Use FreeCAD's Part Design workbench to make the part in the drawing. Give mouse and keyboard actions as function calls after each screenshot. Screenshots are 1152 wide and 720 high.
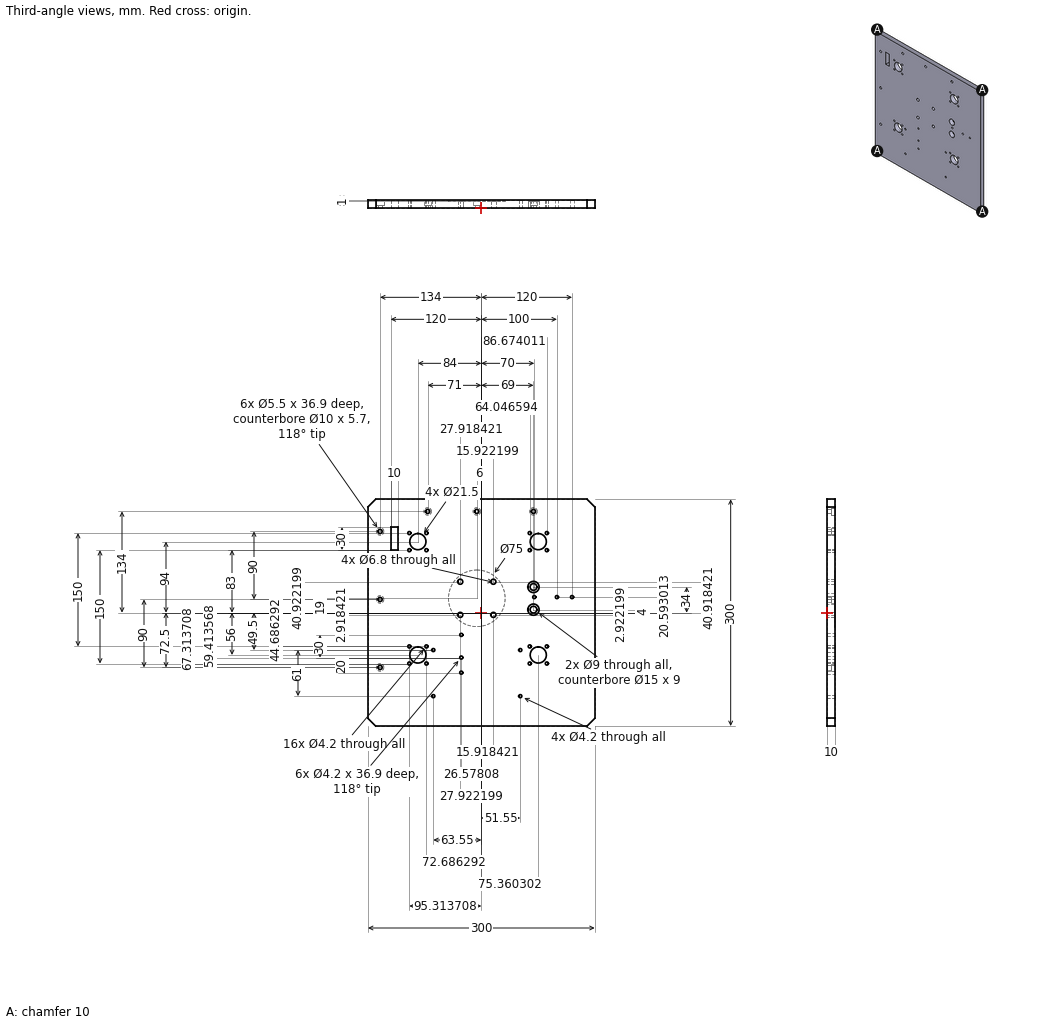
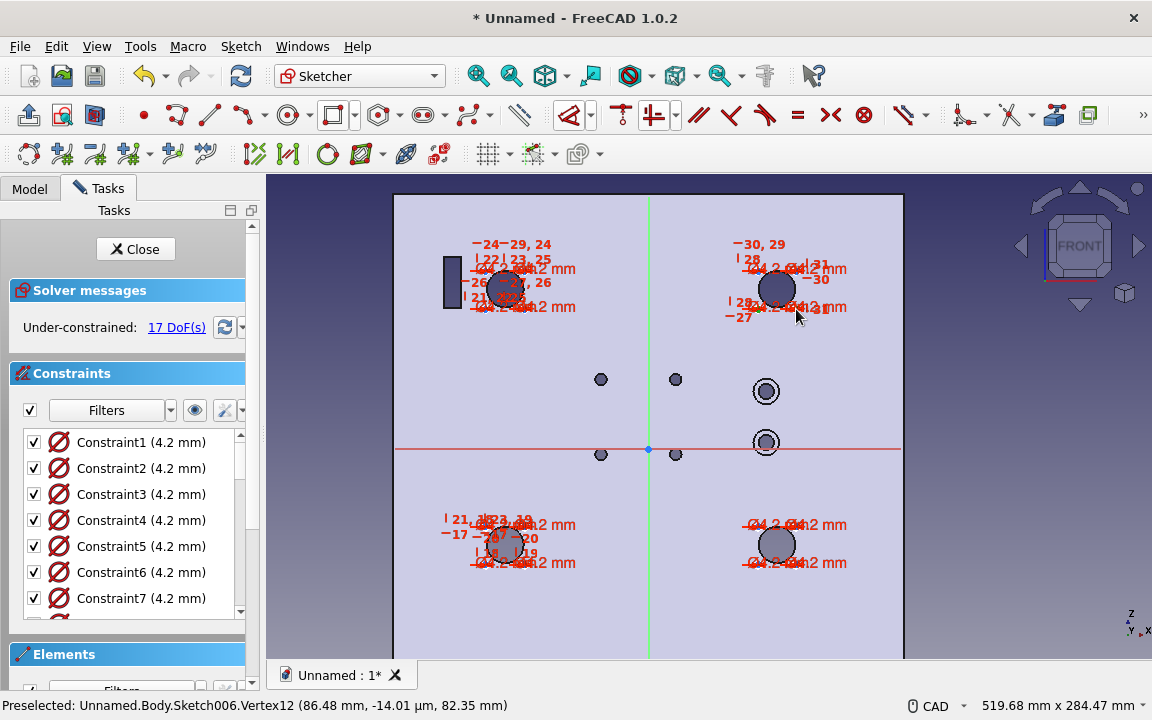
key(h)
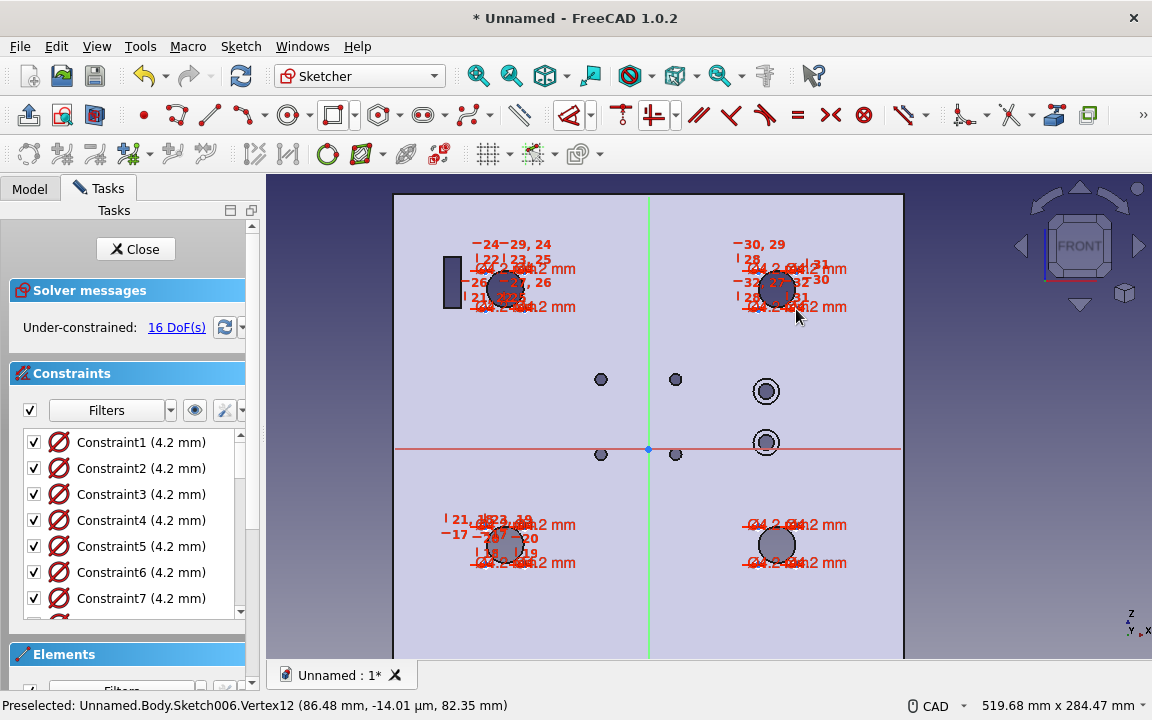
click(758, 309)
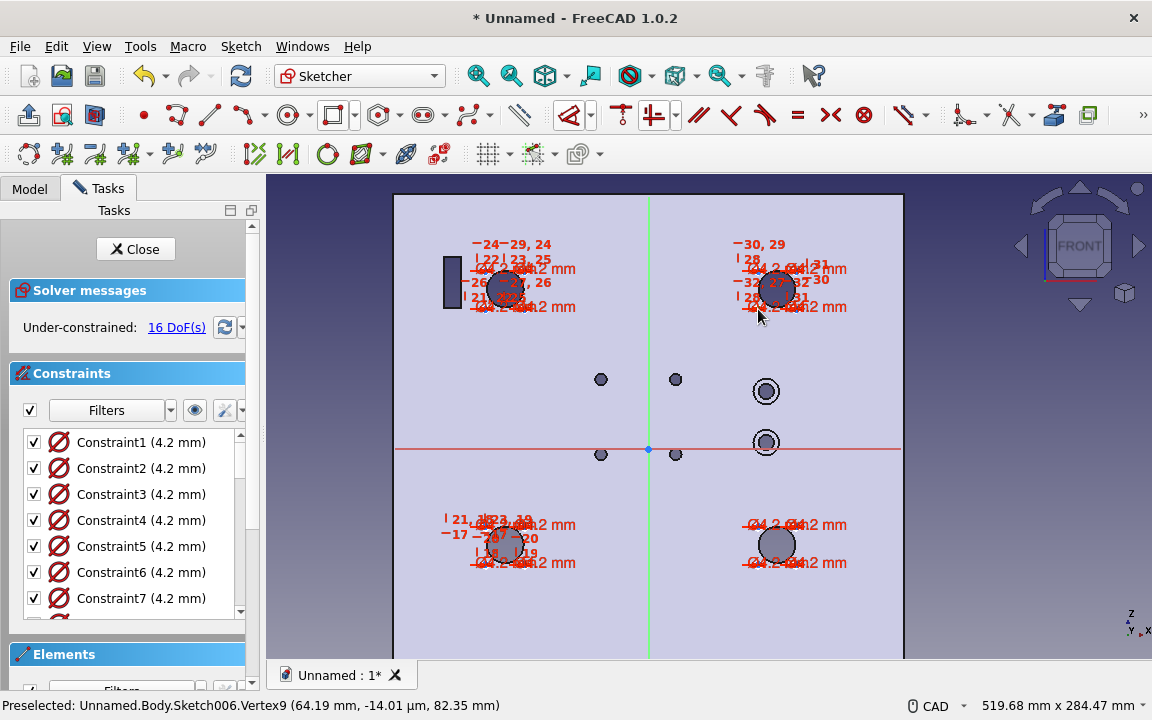
click(758, 565)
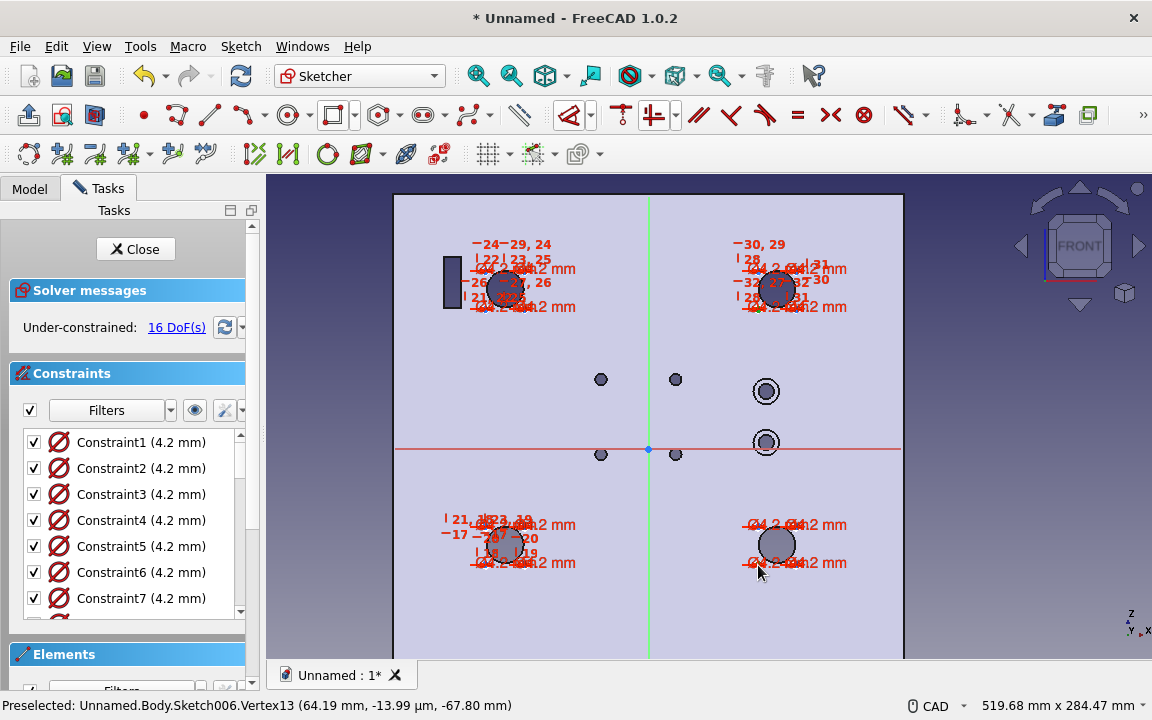
key(v)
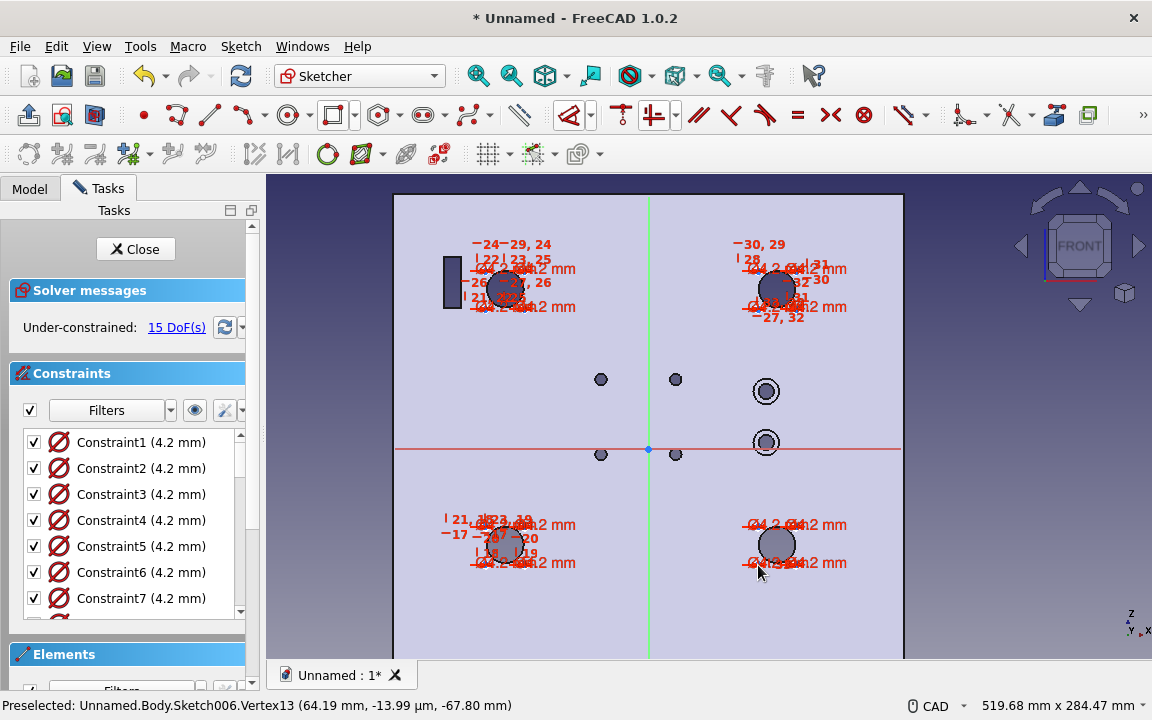
click(525, 565)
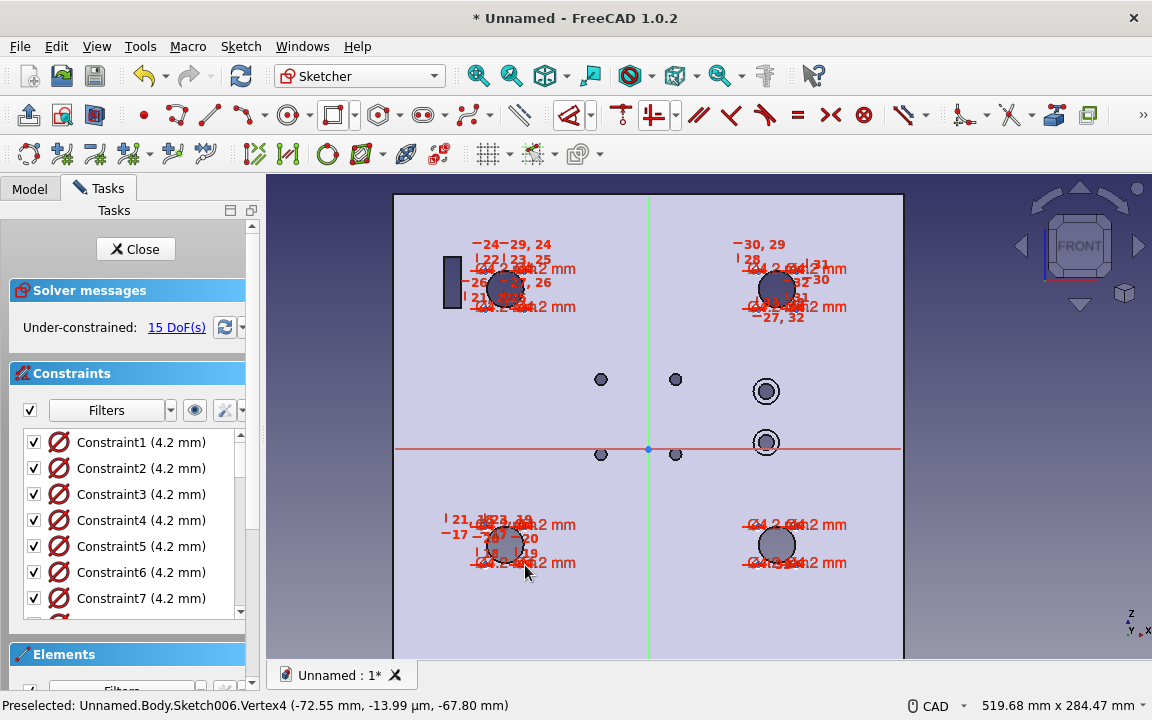
click(758, 565)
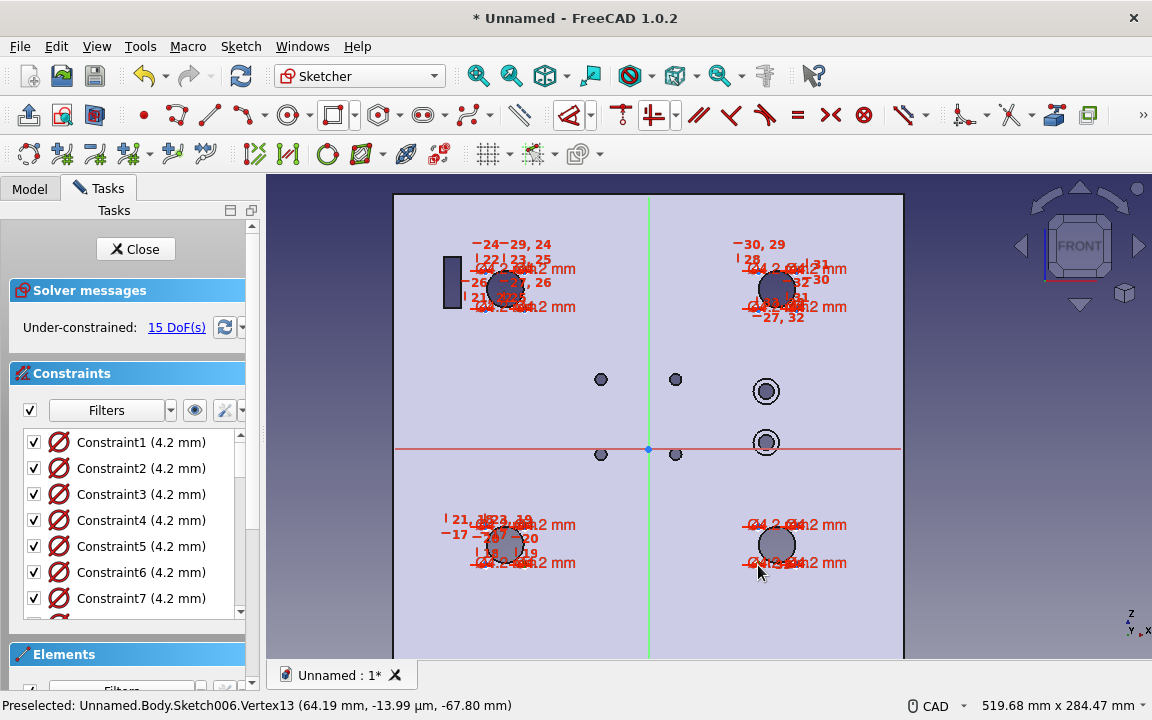
key(h)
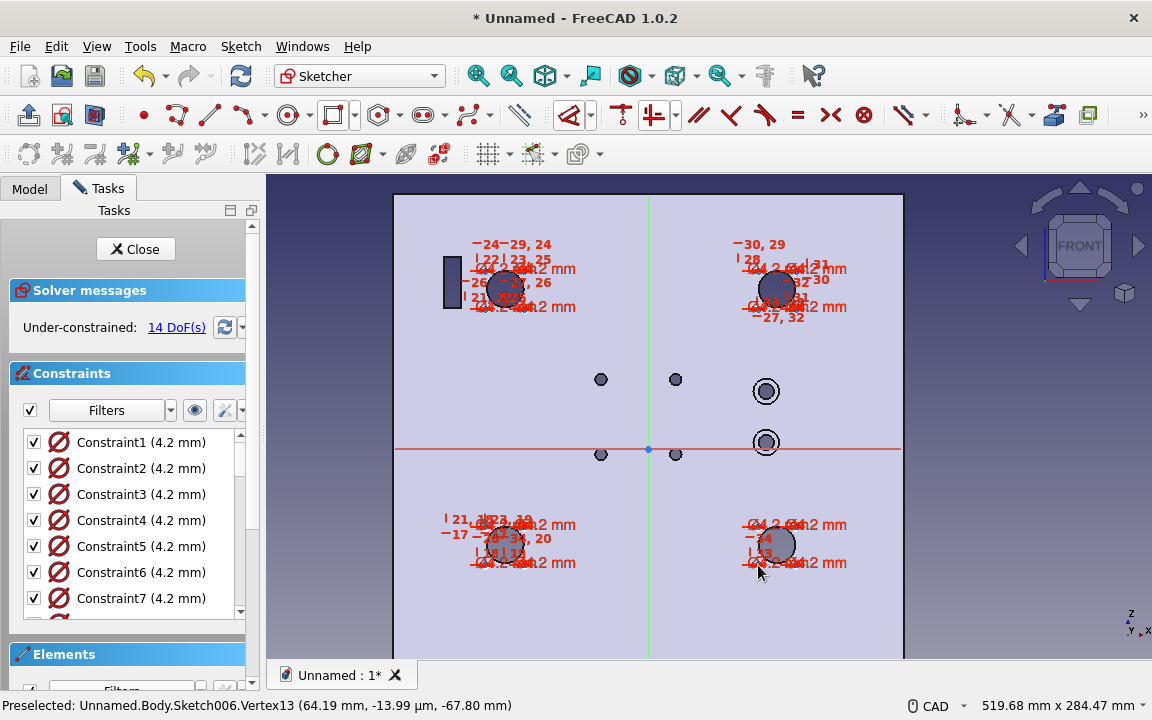
click(758, 565)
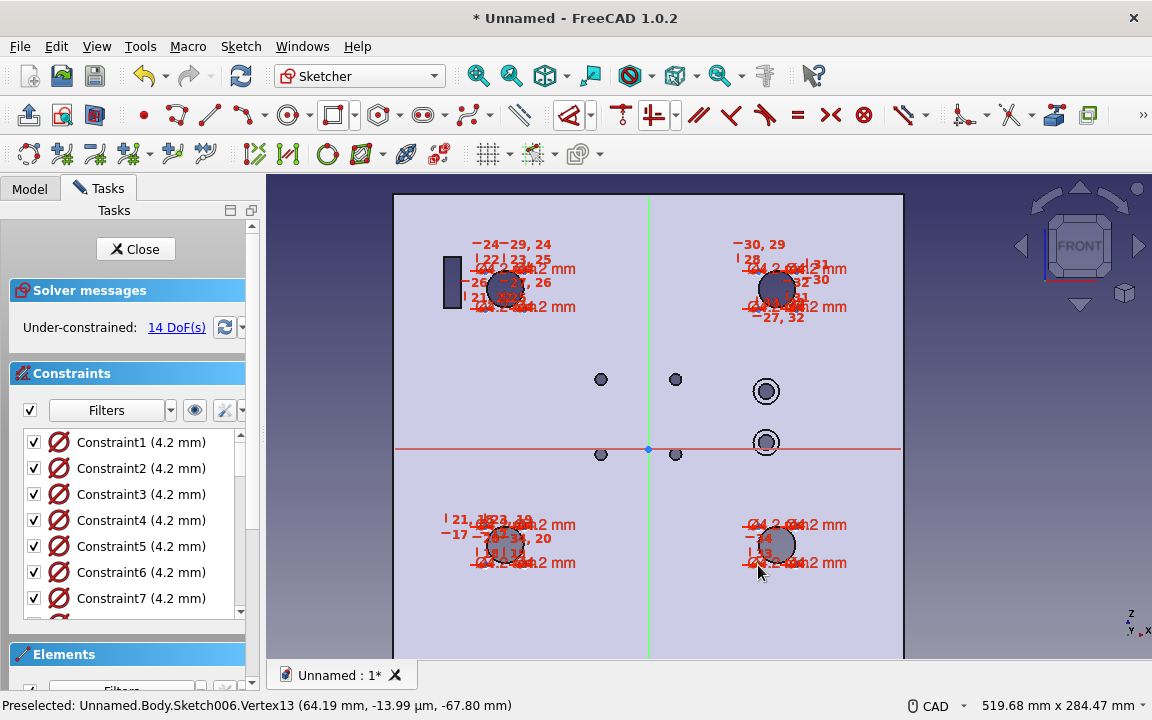
click(758, 527)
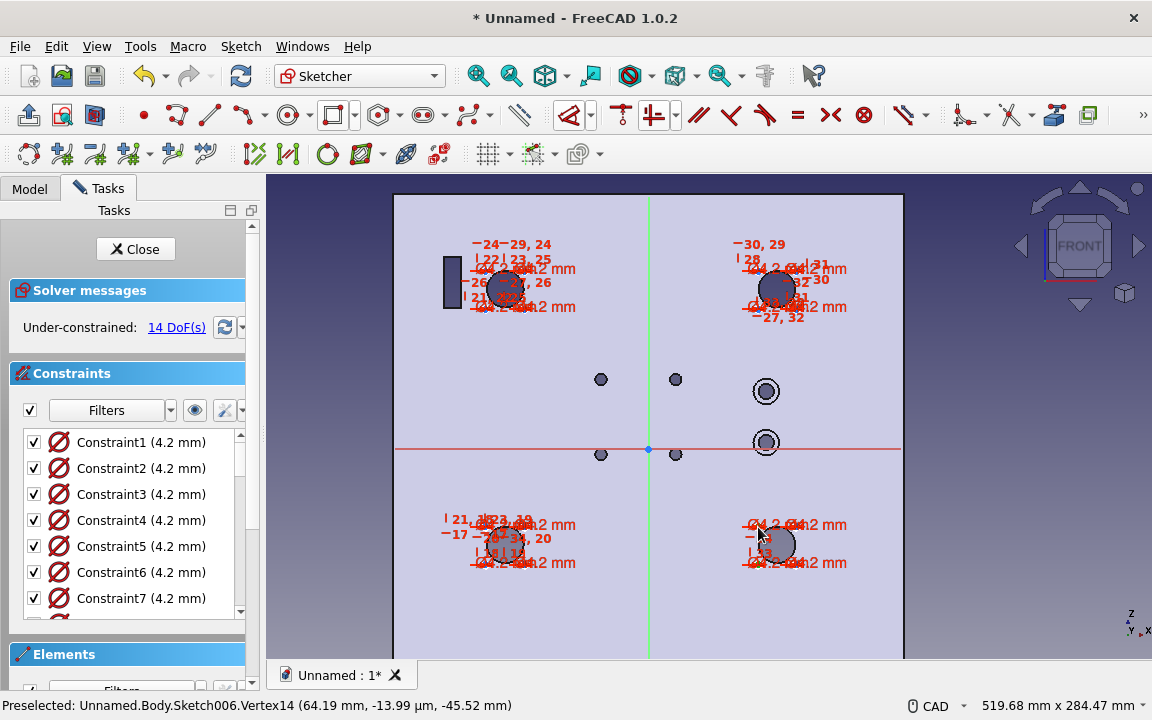
key(v)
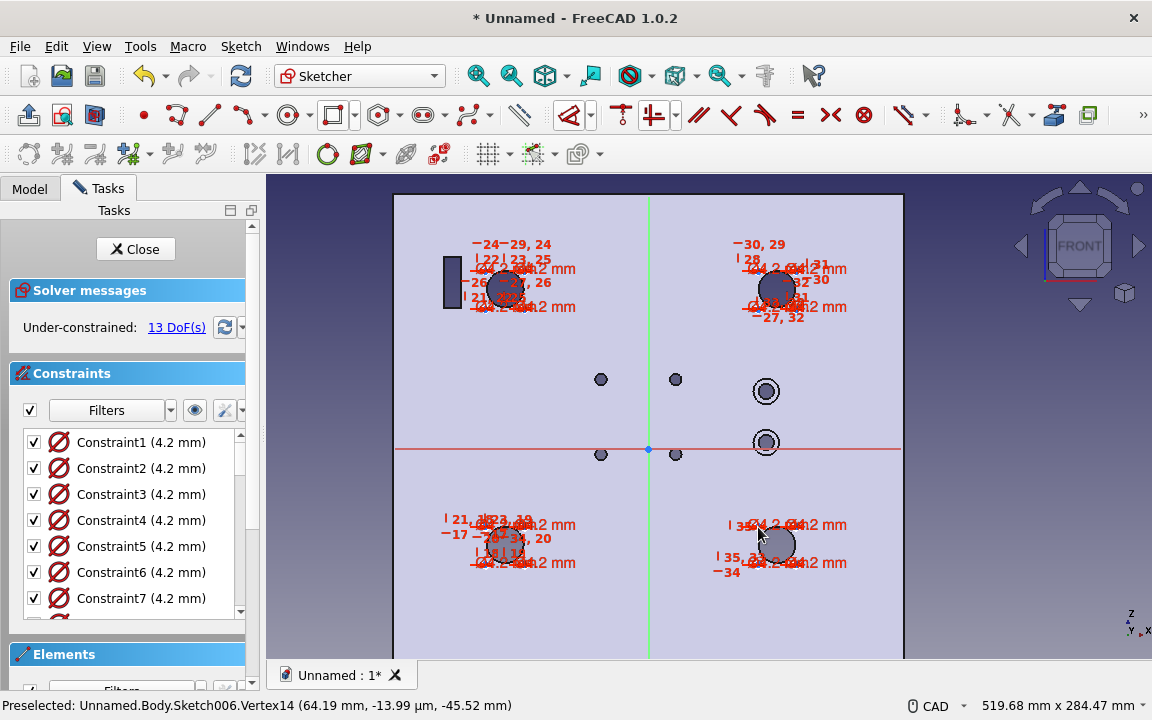
click(525, 527)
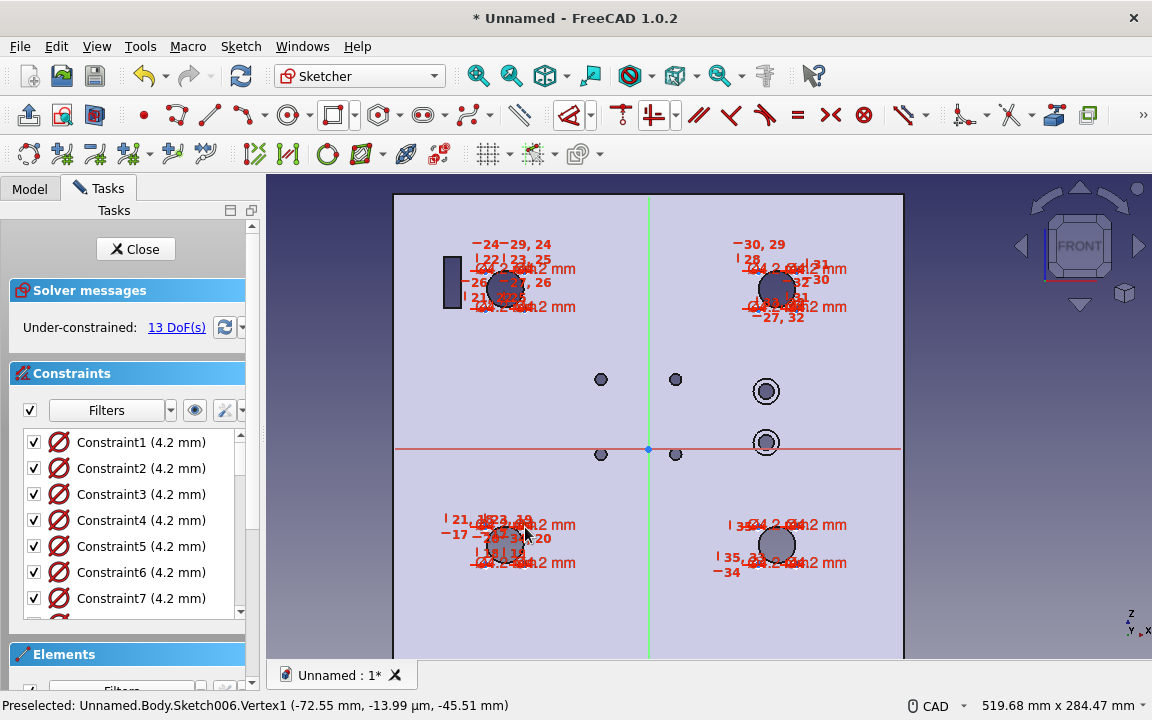
click(758, 527)